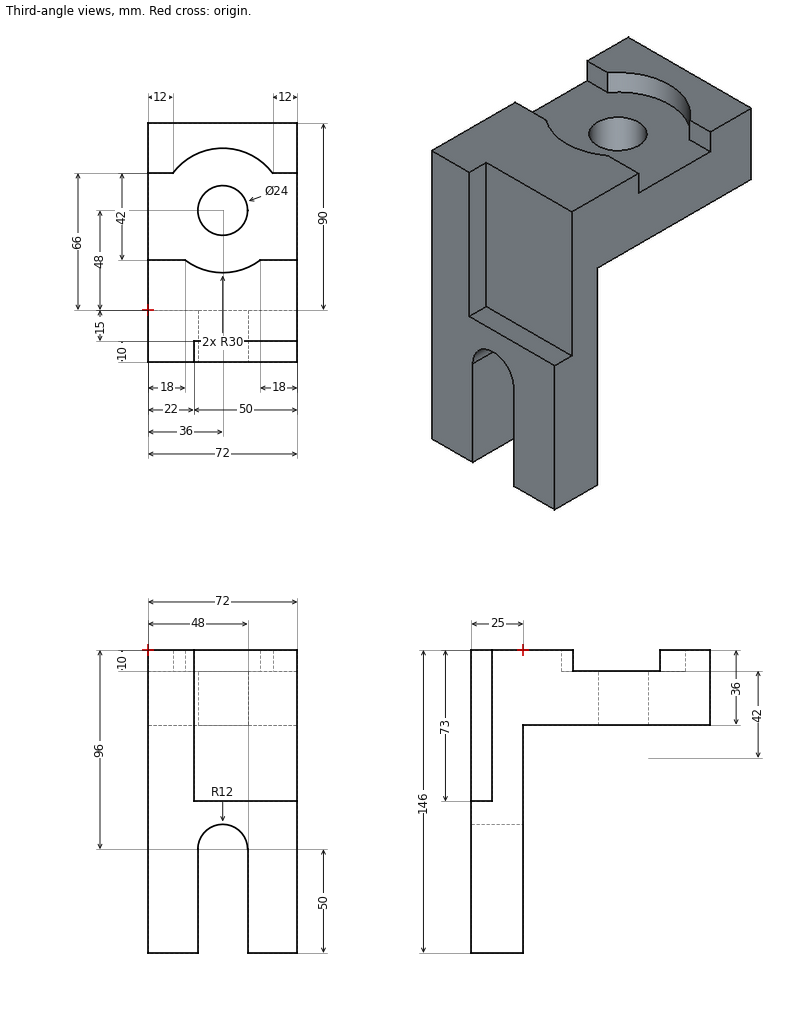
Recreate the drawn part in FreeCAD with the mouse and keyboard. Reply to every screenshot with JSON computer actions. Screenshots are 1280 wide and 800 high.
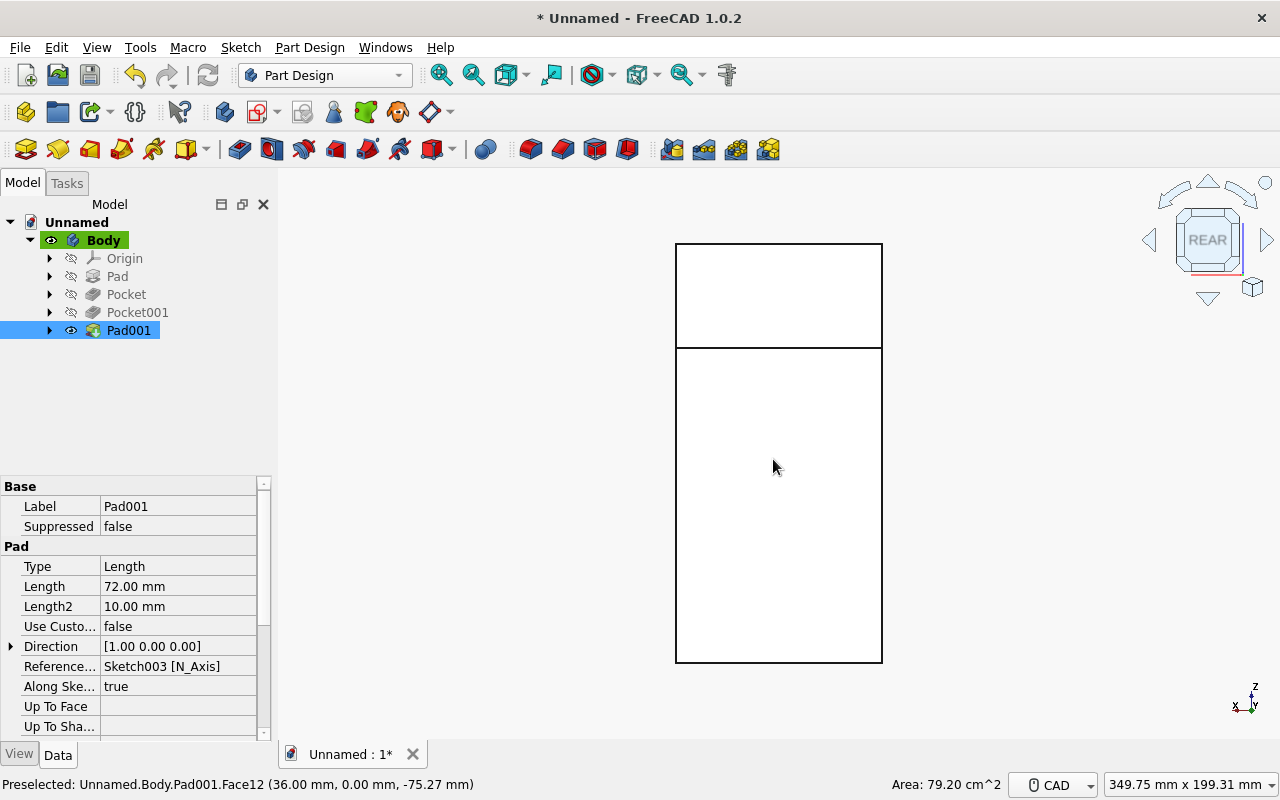
{"action": "left_click", "coordinate": [258, 112]}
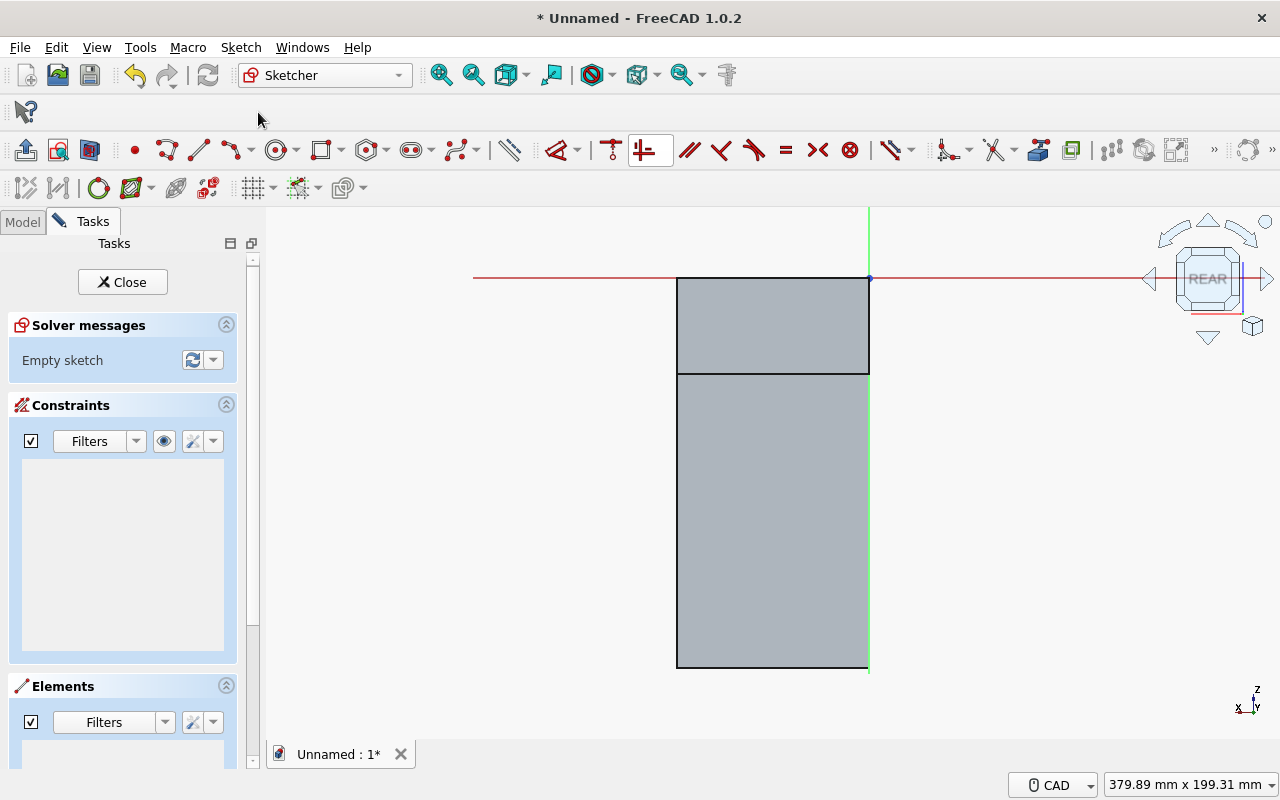
{"action": "left_click", "coordinate": [168, 150]}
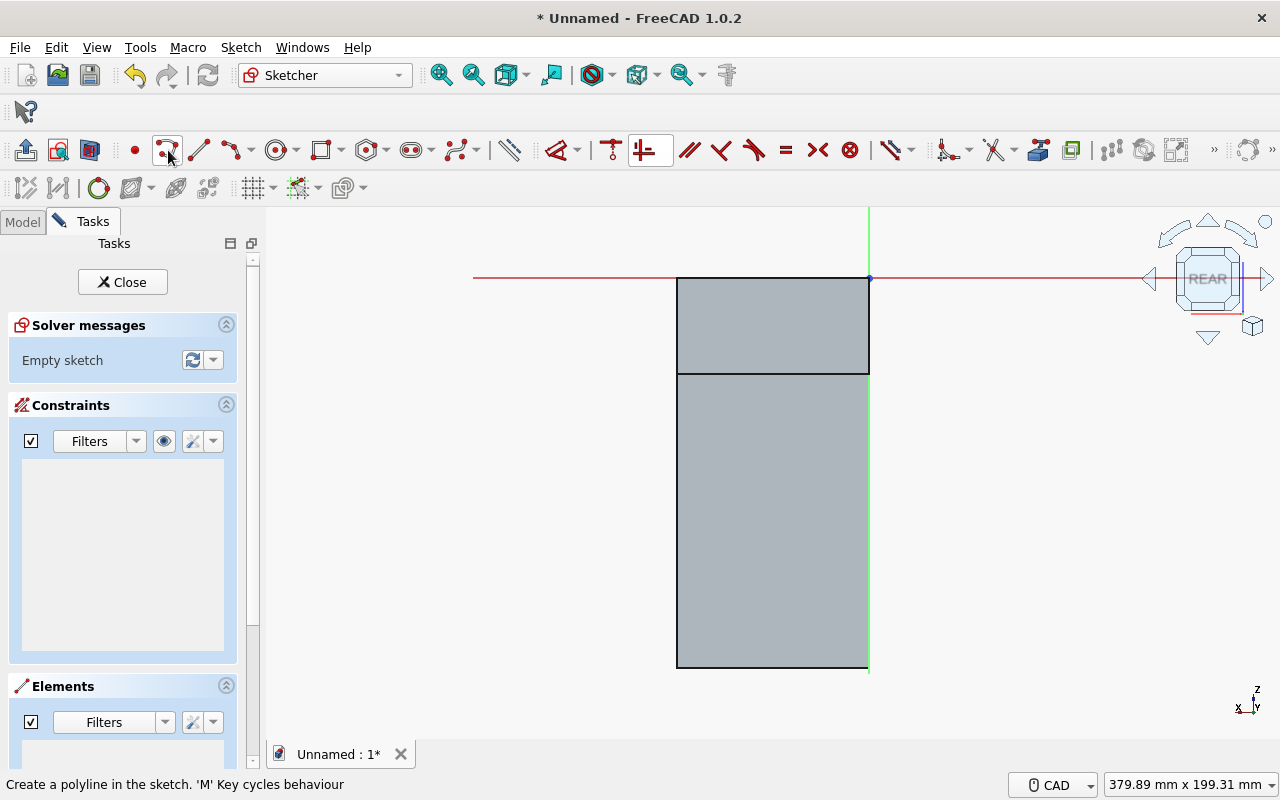
{"action": "left_click", "coordinate": [741, 534]}
{"action": "left_click", "coordinate": [741, 668]}
{"action": "left_click", "coordinate": [805, 668]}
{"action": "left_click", "coordinate": [805, 534]}
{"action": "right_click", "coordinate": [805, 534]}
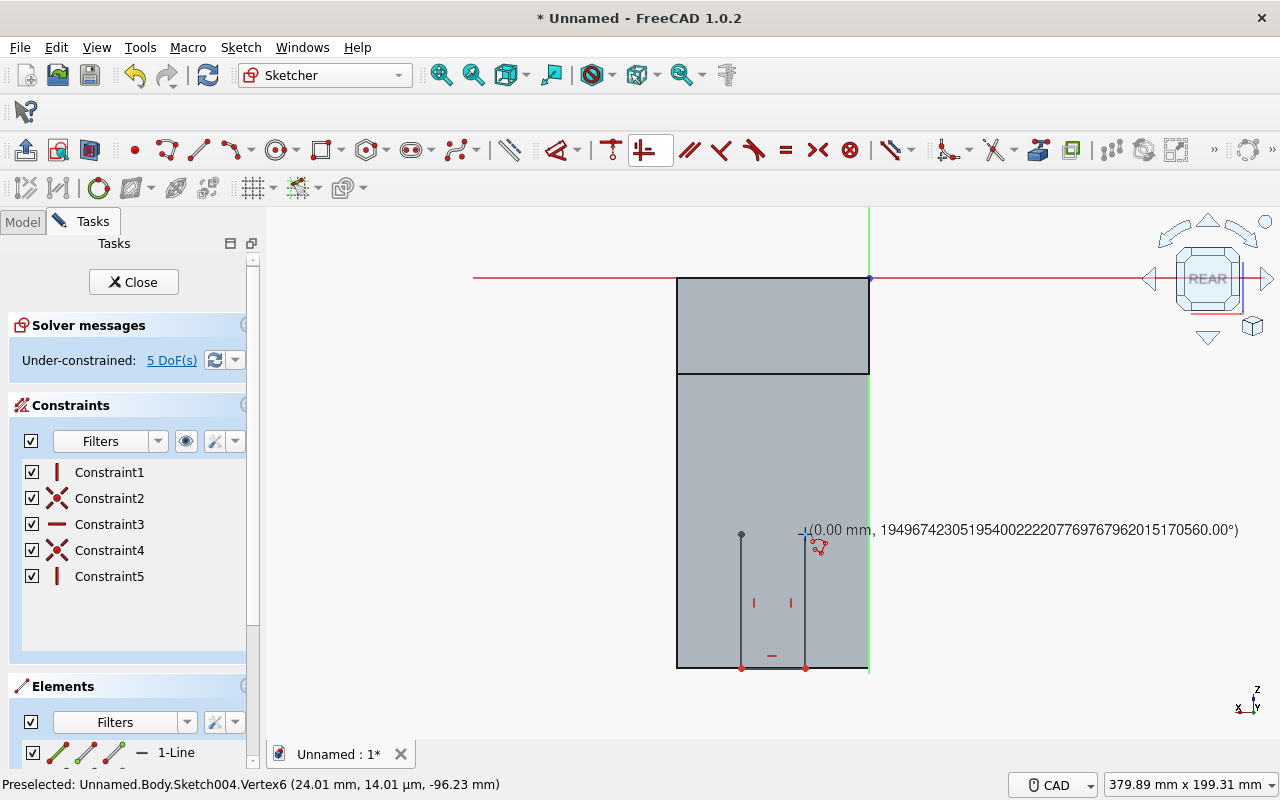
{"action": "key", "text": "g 3 a"}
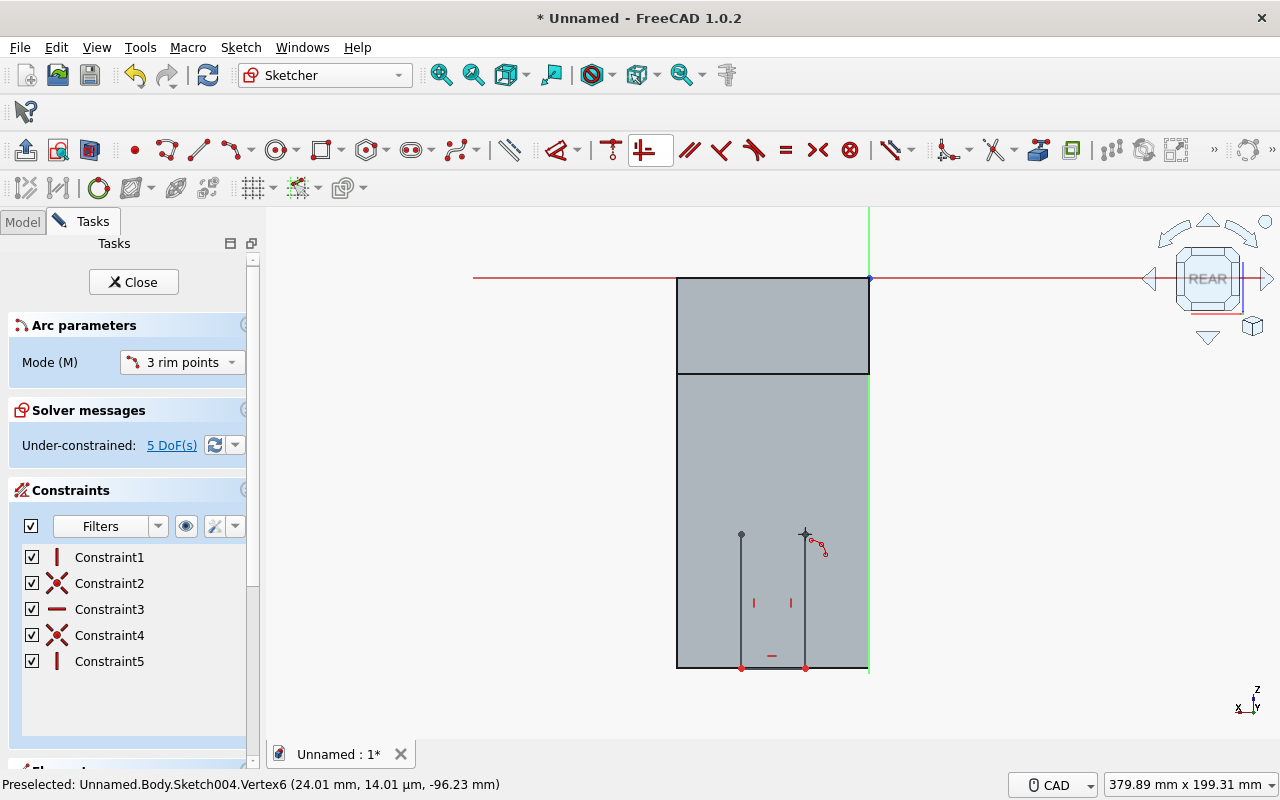
{"action": "left_click", "coordinate": [805, 535]}
{"action": "left_click", "coordinate": [741, 535]}
{"action": "left_click", "coordinate": [773, 502]}
{"action": "key", "text": "Escape"}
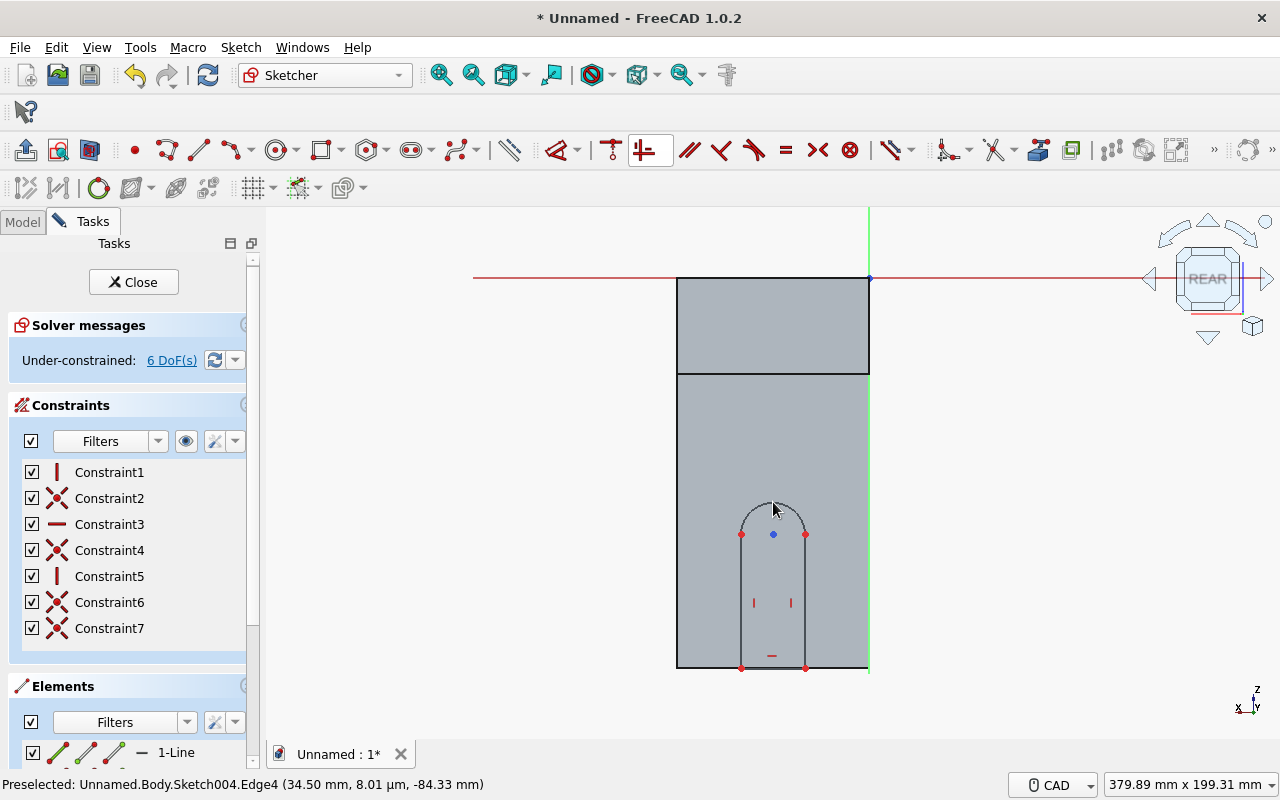
{"action": "left_click", "coordinate": [741, 575]}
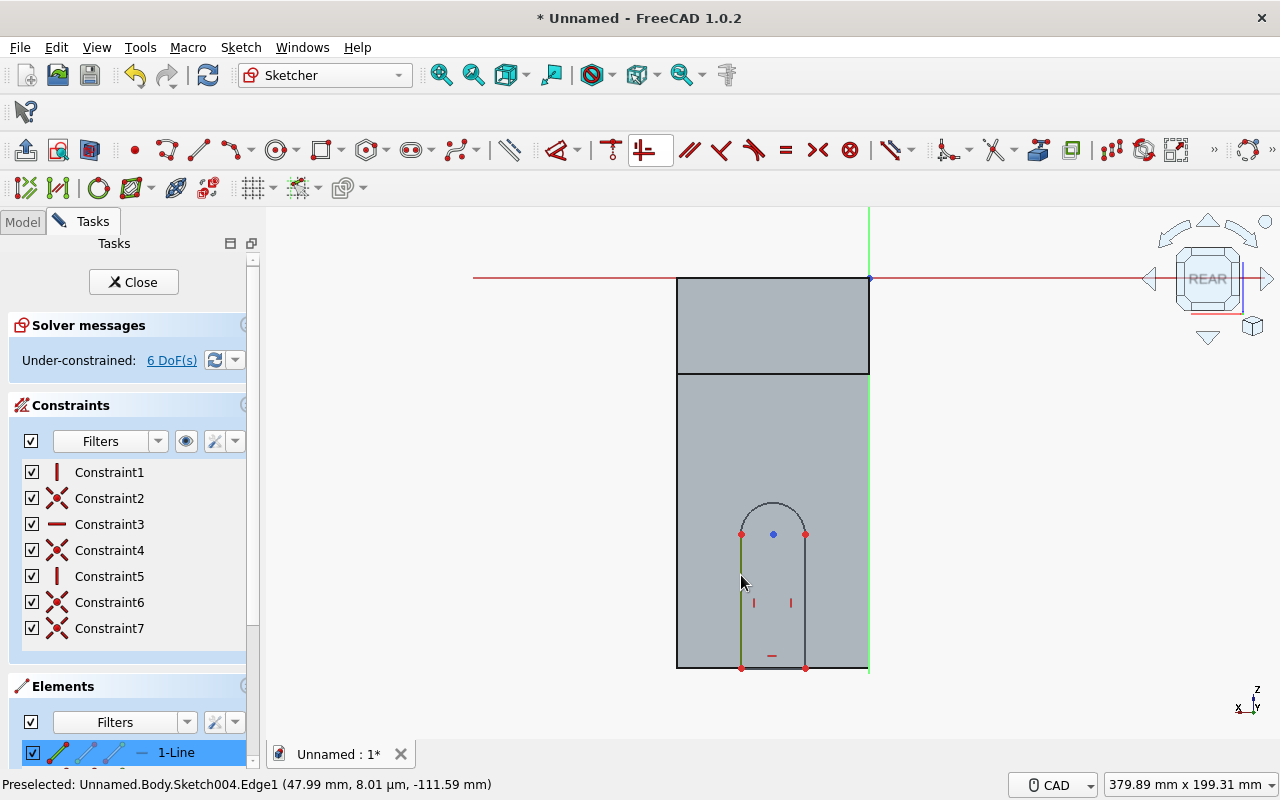
{"action": "left_click", "coordinate": [792, 509]}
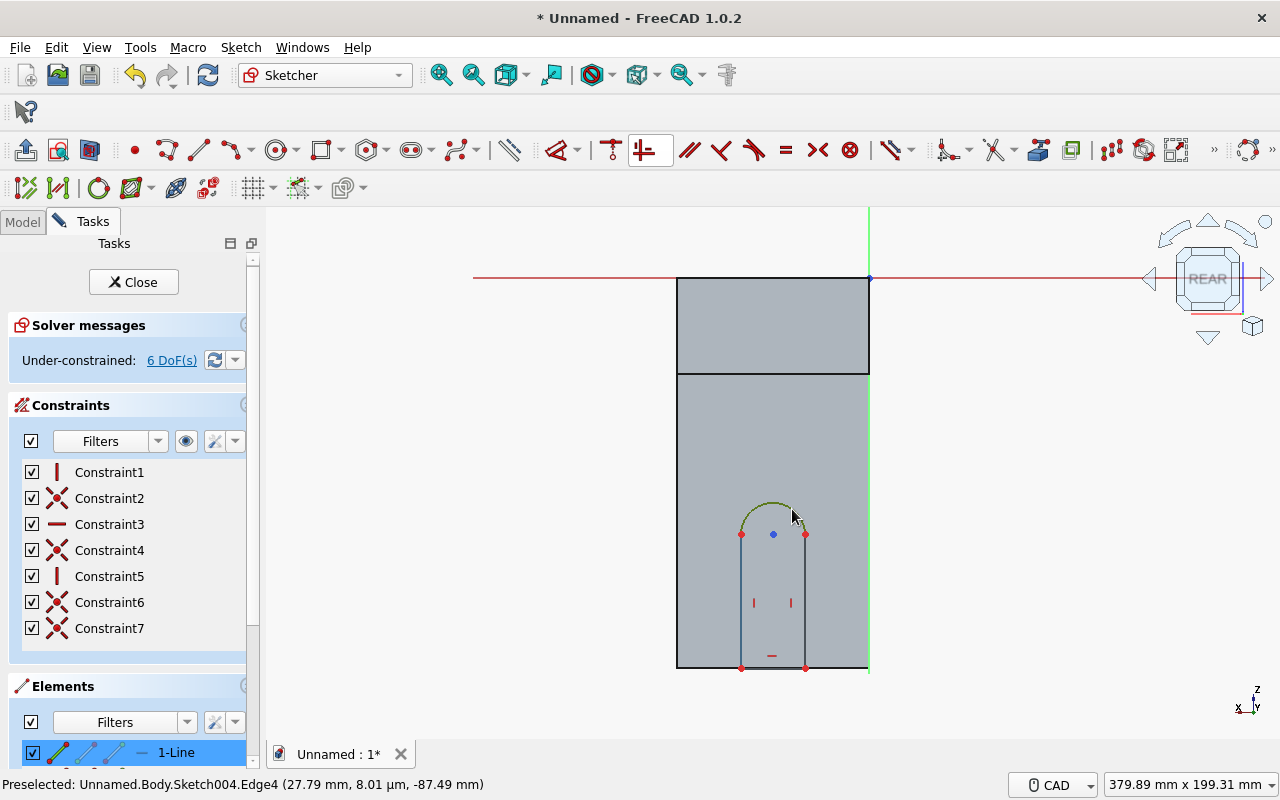
{"action": "left_click", "coordinate": [754, 150]}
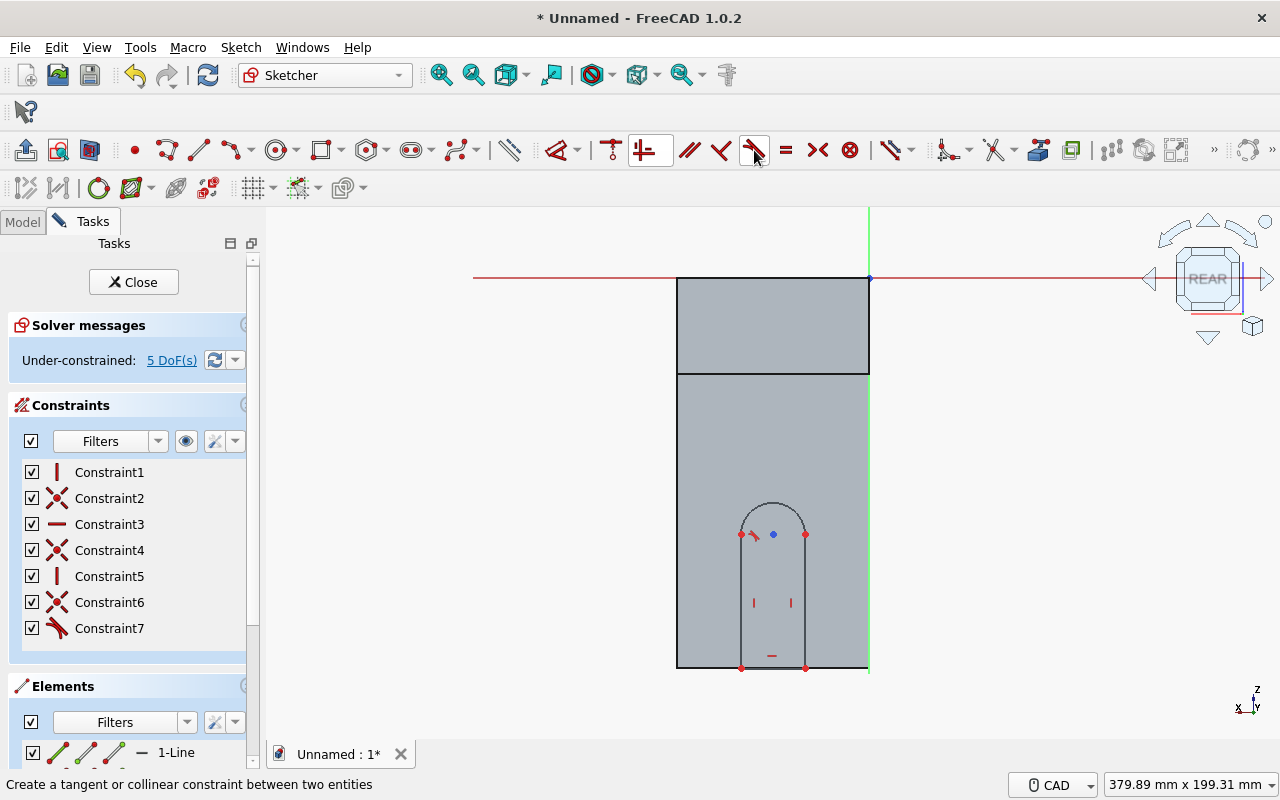
{"action": "left_click", "coordinate": [805, 629]}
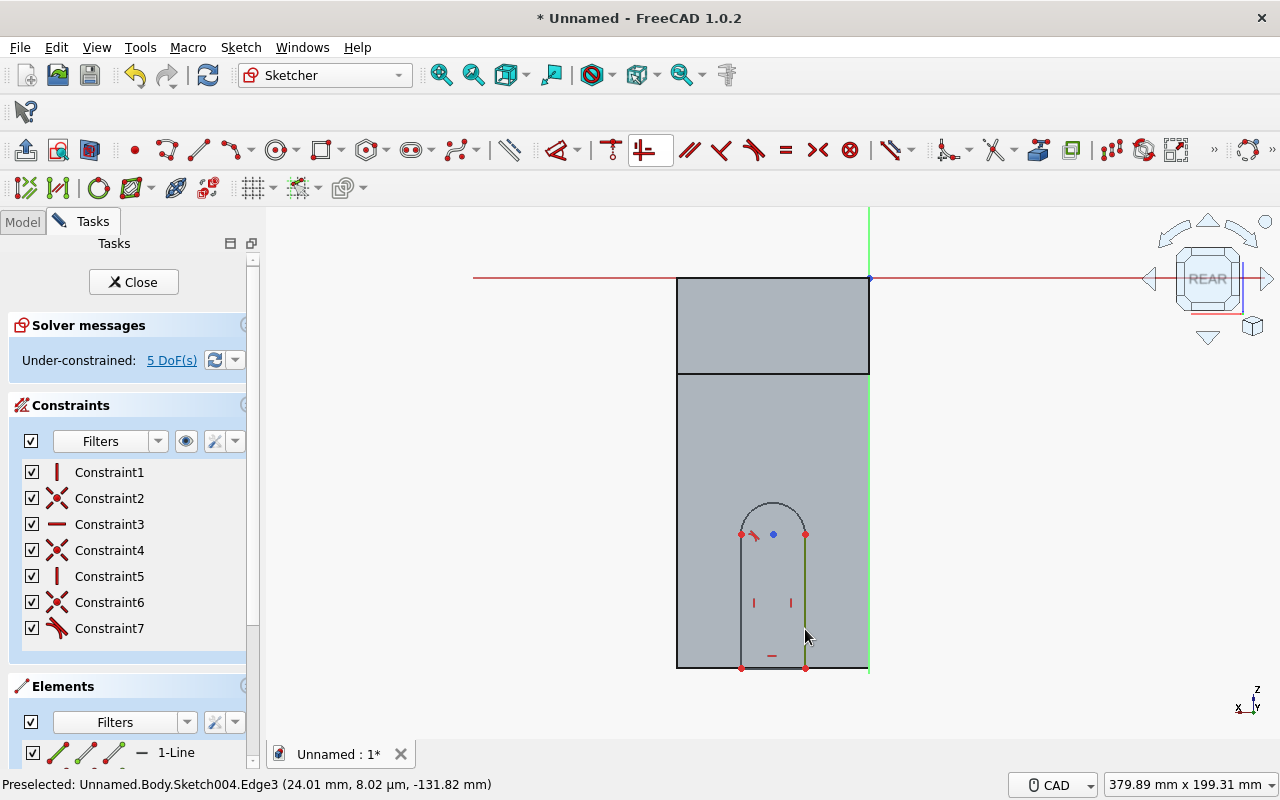
{"action": "left_click", "coordinate": [792, 509]}